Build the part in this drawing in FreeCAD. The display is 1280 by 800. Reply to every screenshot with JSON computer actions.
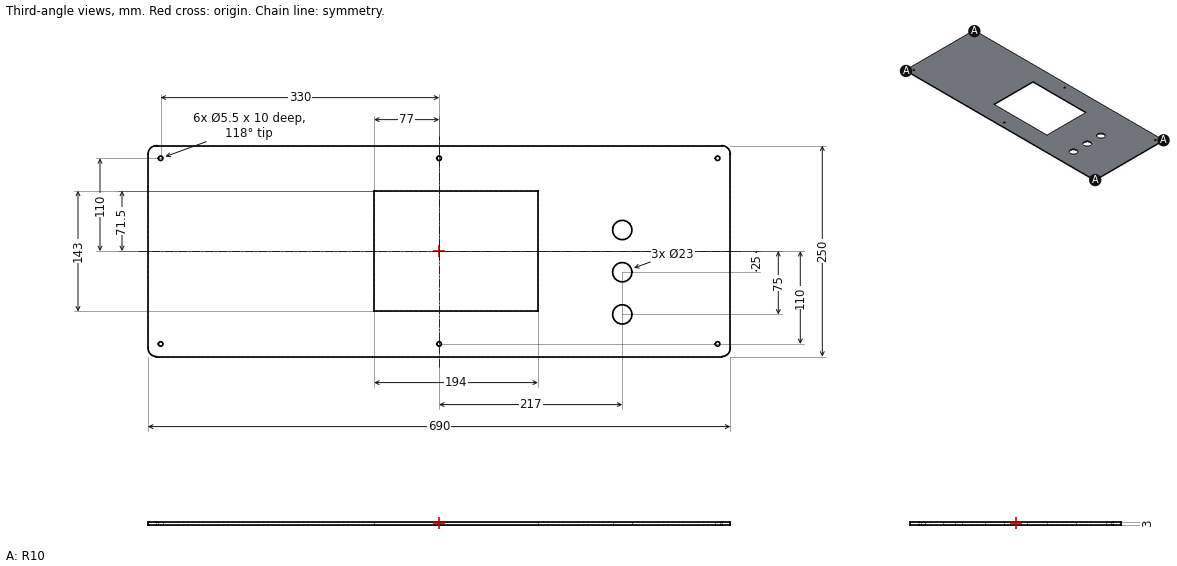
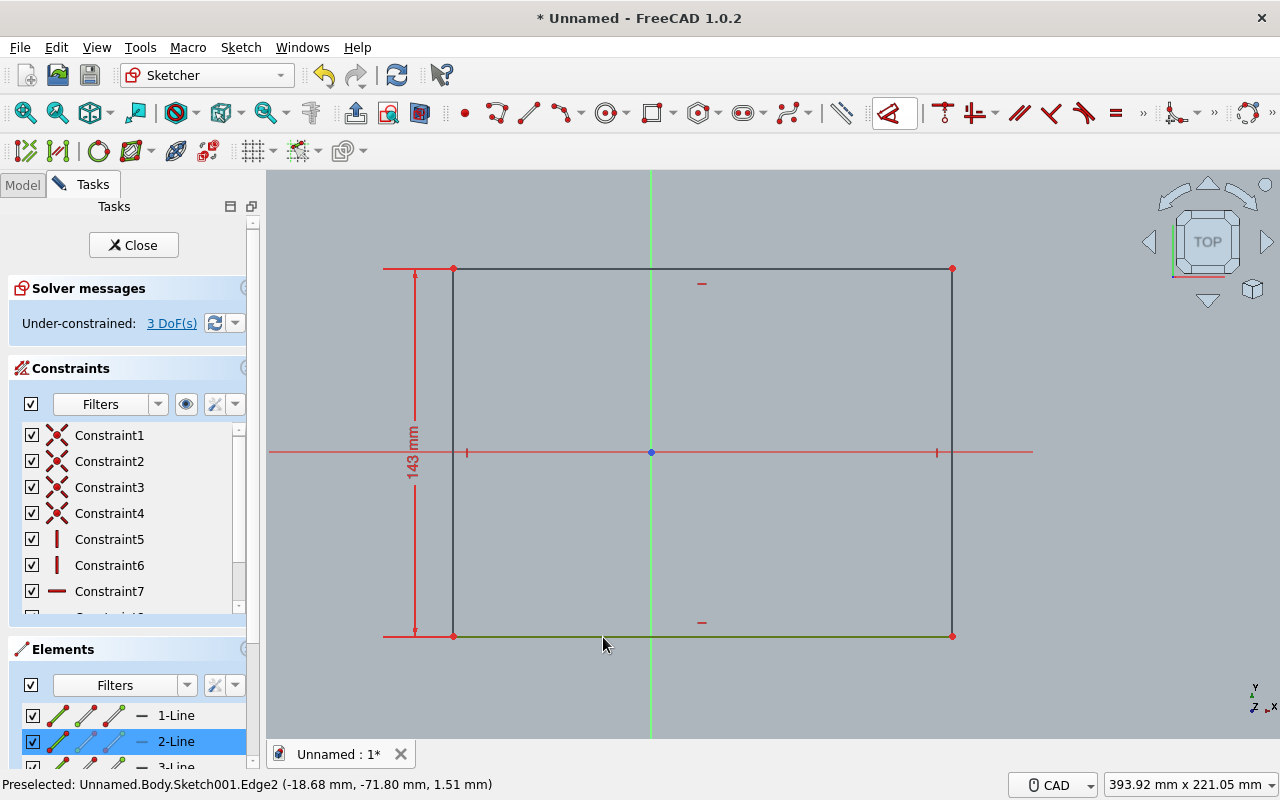
{"action": "left_click", "coordinate": [912, 114]}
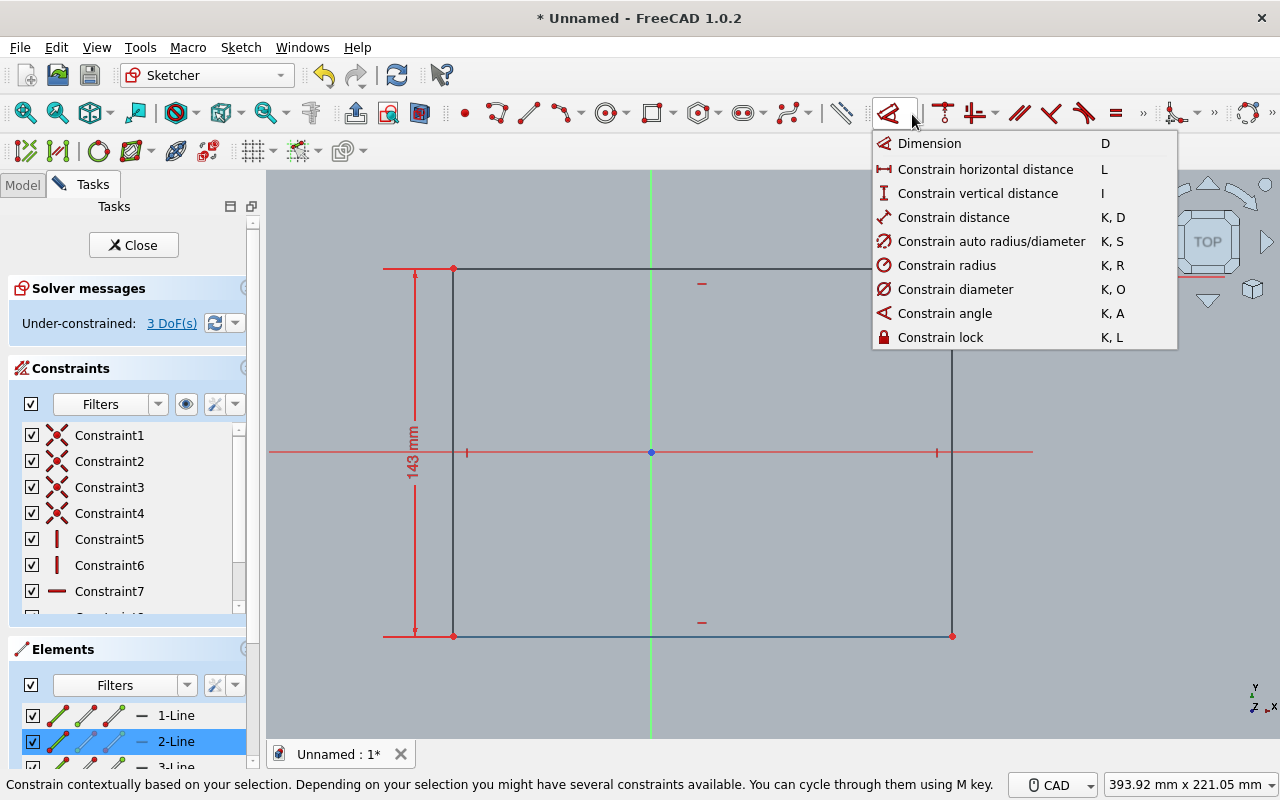
{"action": "left_click", "coordinate": [1025, 169]}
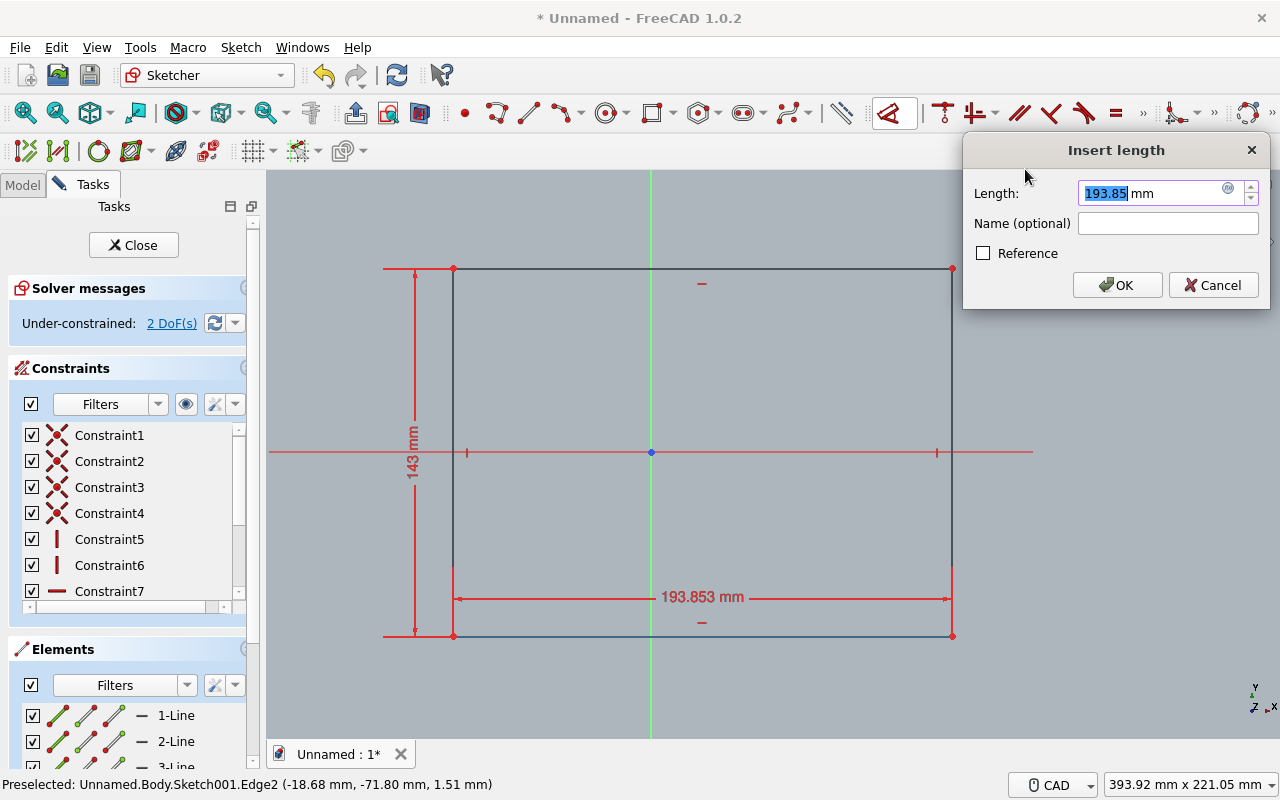
{"action": "type", "text": "194"}
{"action": "key", "text": "Return"}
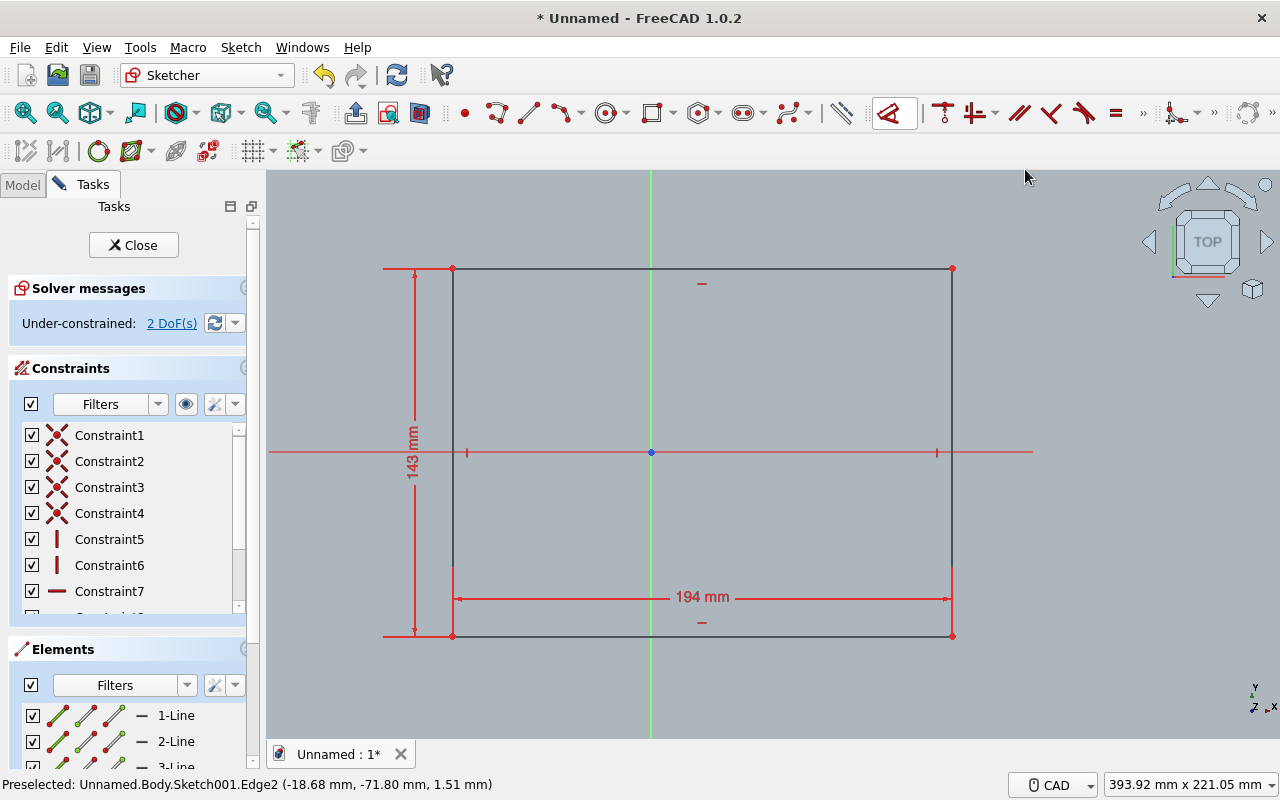
{"action": "left_click", "coordinate": [453, 269]}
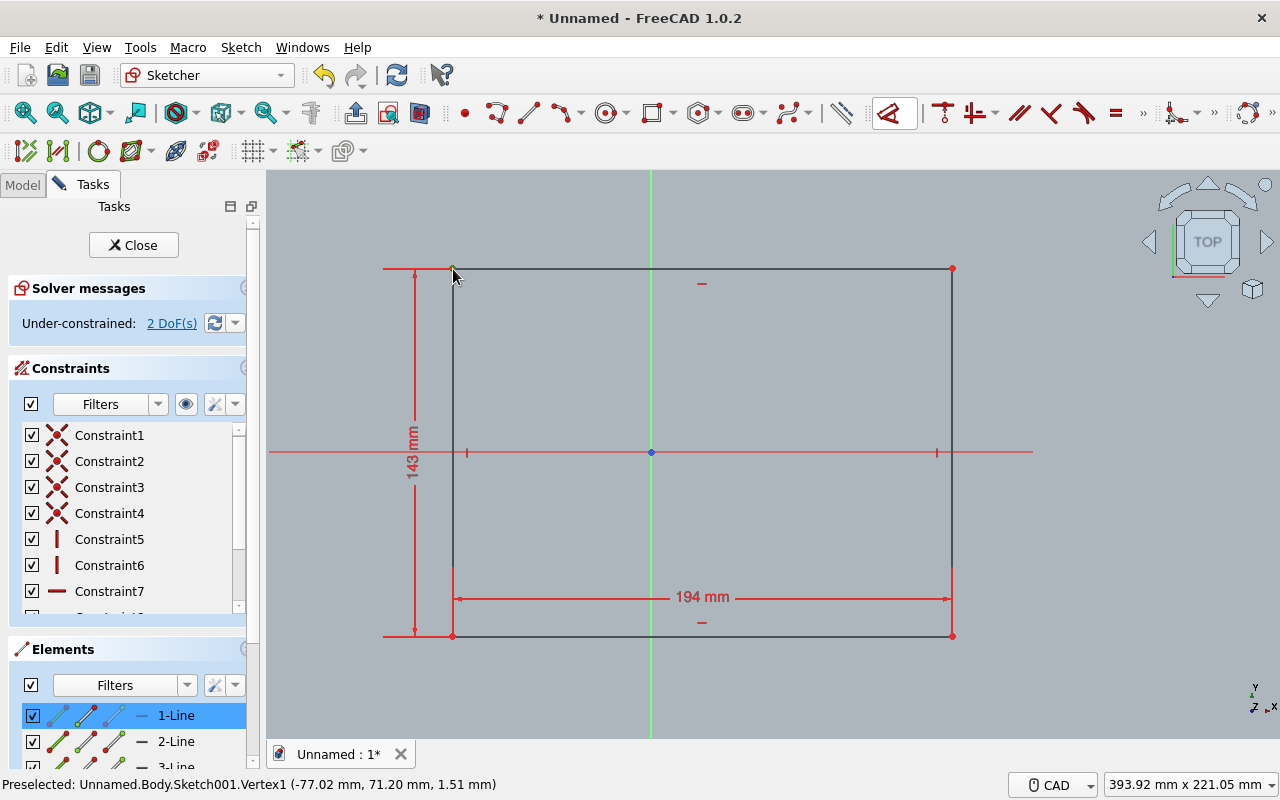
{"action": "left_click", "coordinate": [912, 114]}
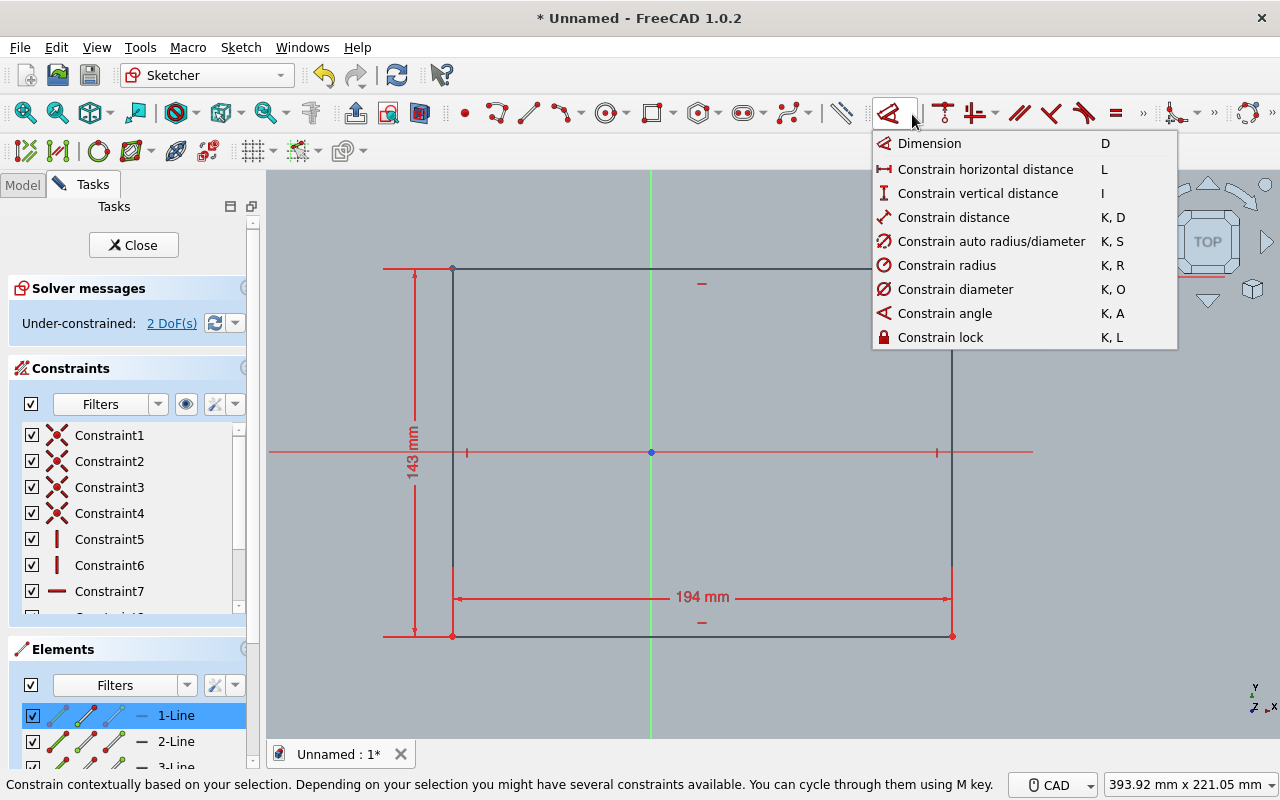
{"action": "left_click", "coordinate": [1025, 169]}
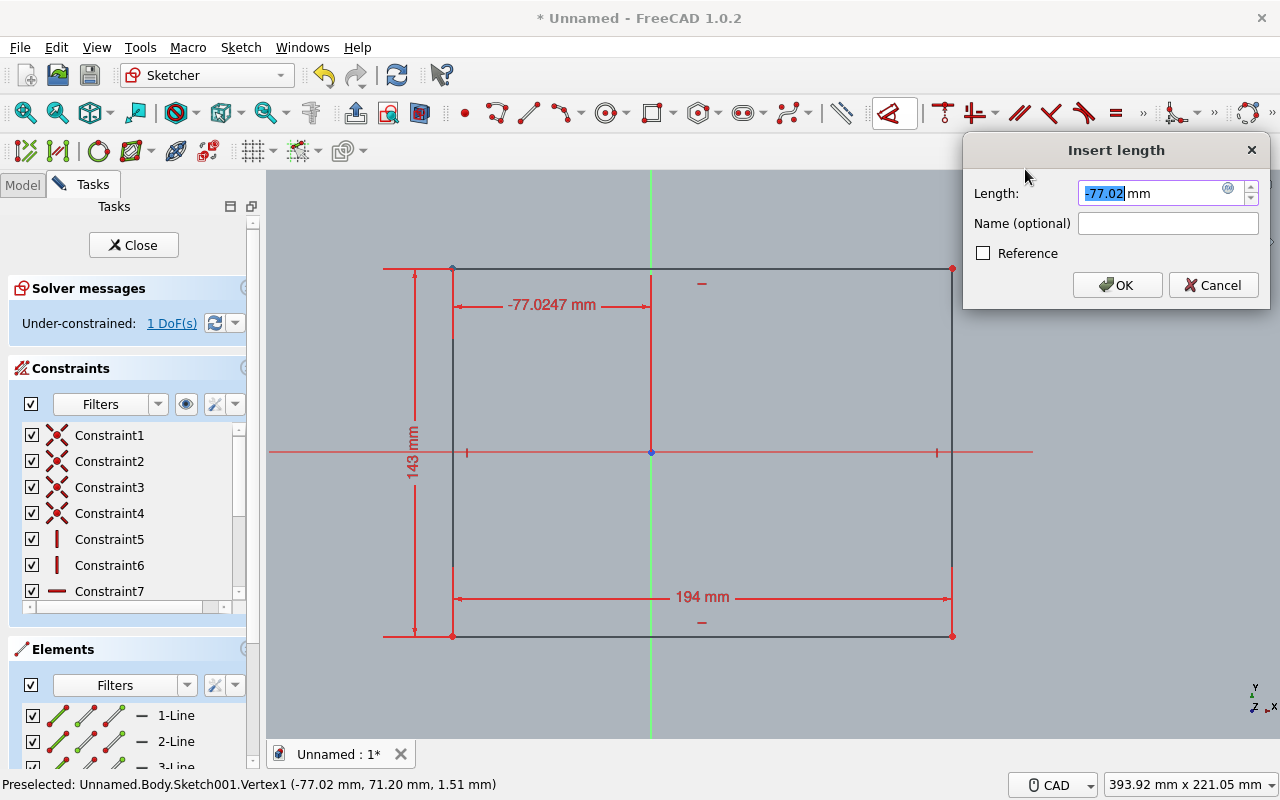
{"action": "type", "text": "-77"}
{"action": "key", "text": "Return"}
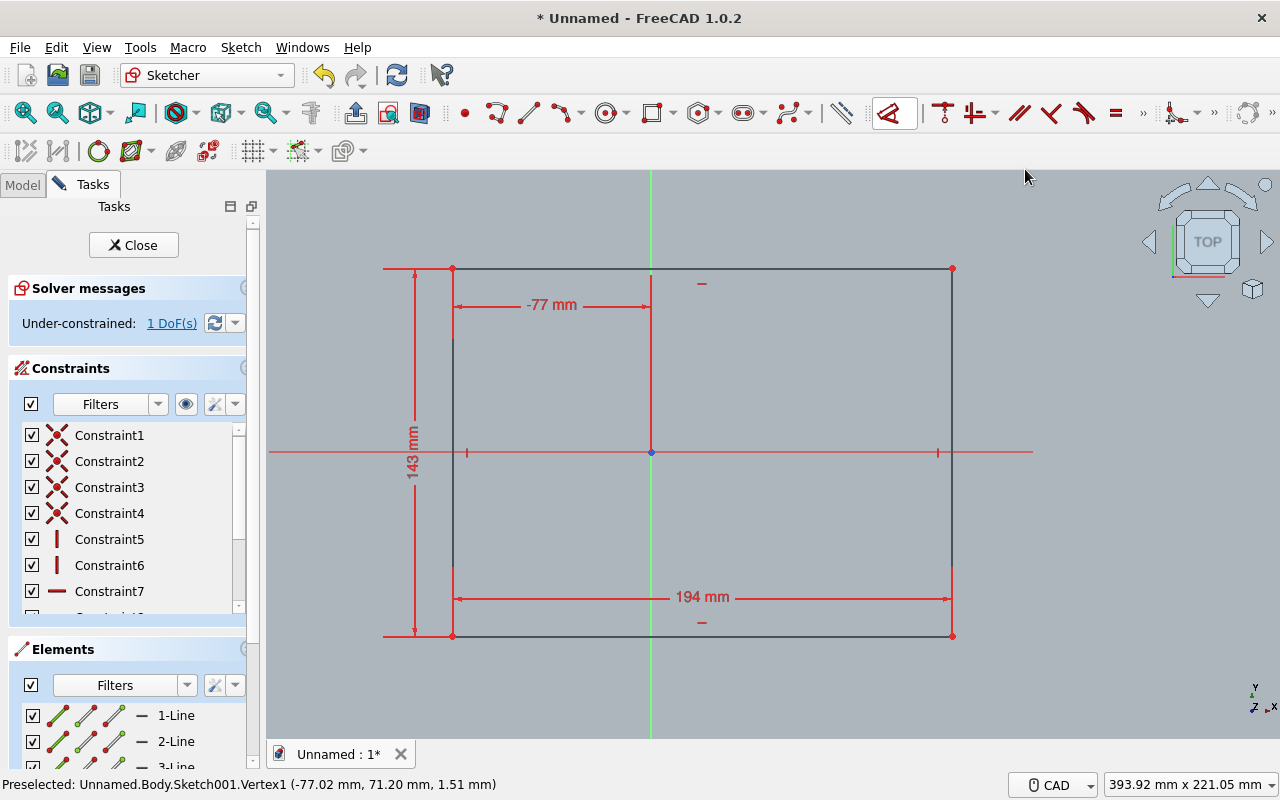
{"action": "left_click", "coordinate": [453, 269]}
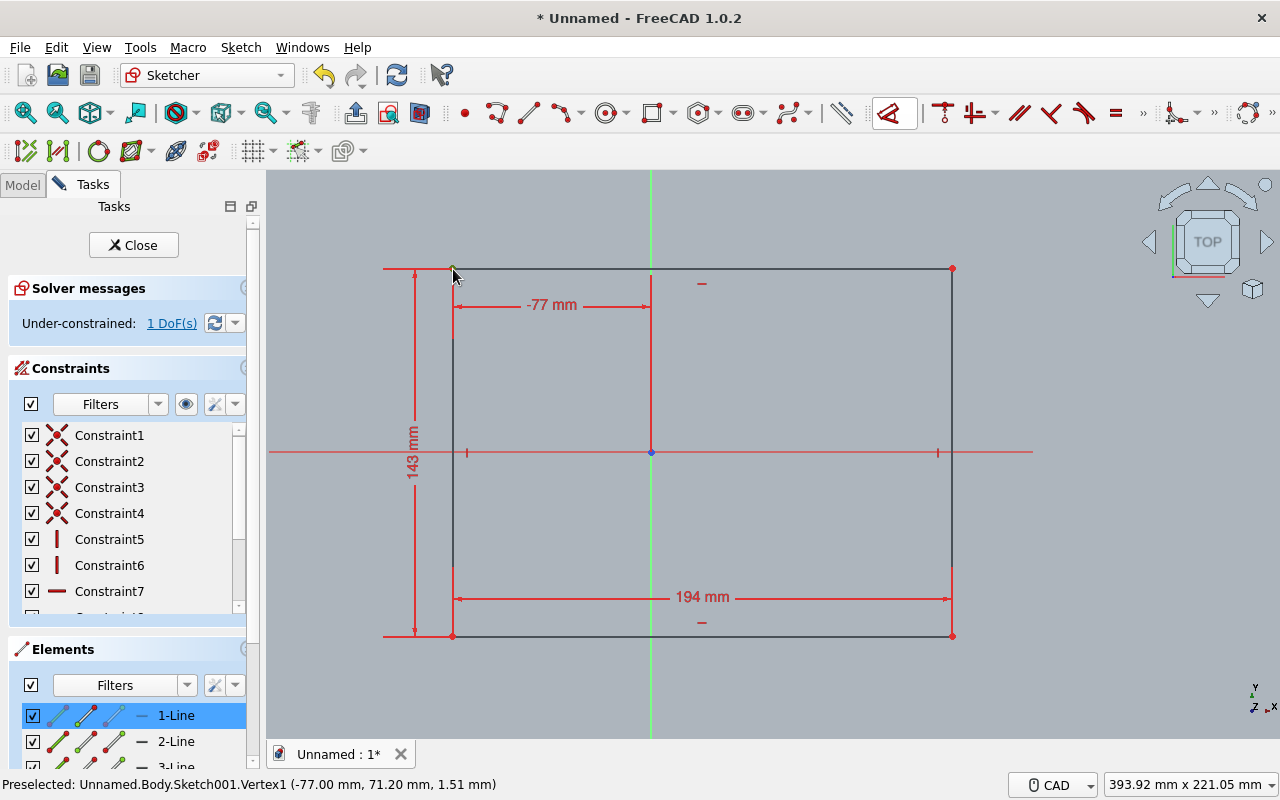
{"action": "key", "text": "i"}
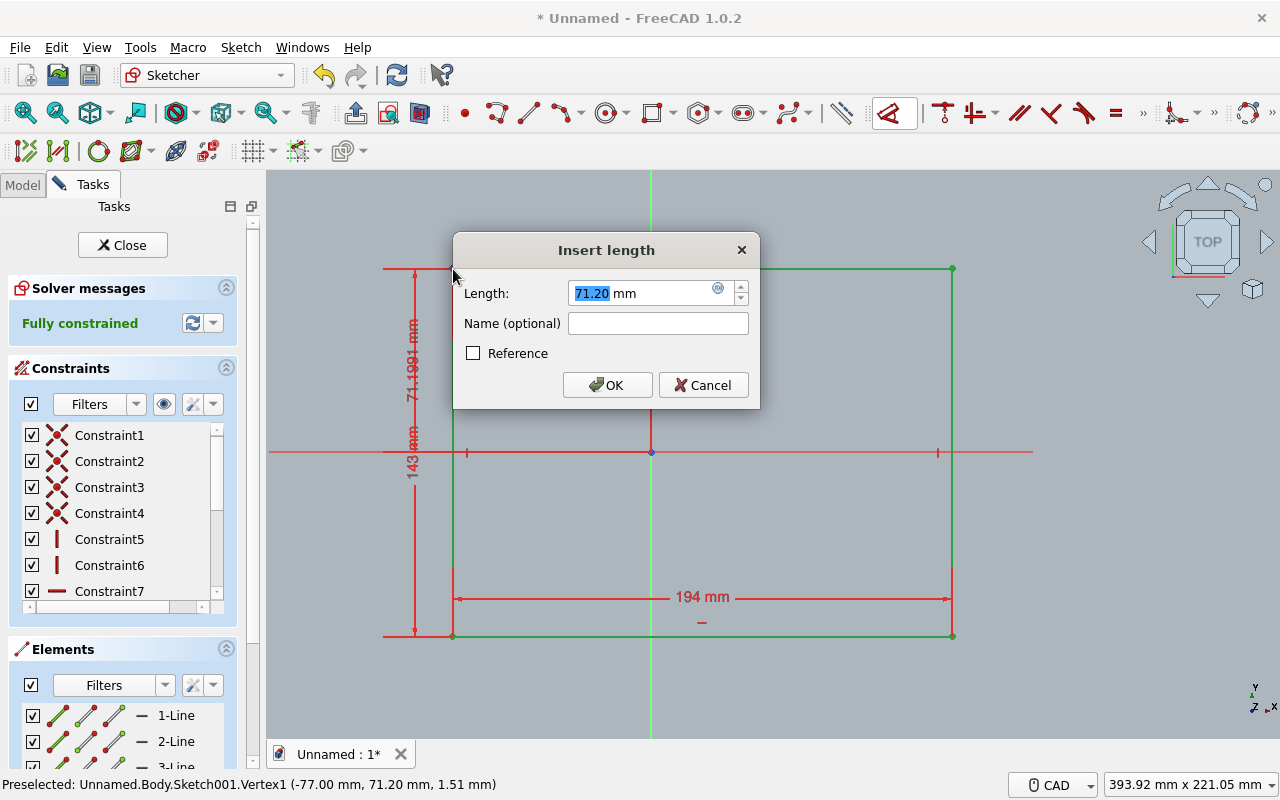
{"action": "type", "text": "71.5"}
{"action": "key", "text": "Return"}